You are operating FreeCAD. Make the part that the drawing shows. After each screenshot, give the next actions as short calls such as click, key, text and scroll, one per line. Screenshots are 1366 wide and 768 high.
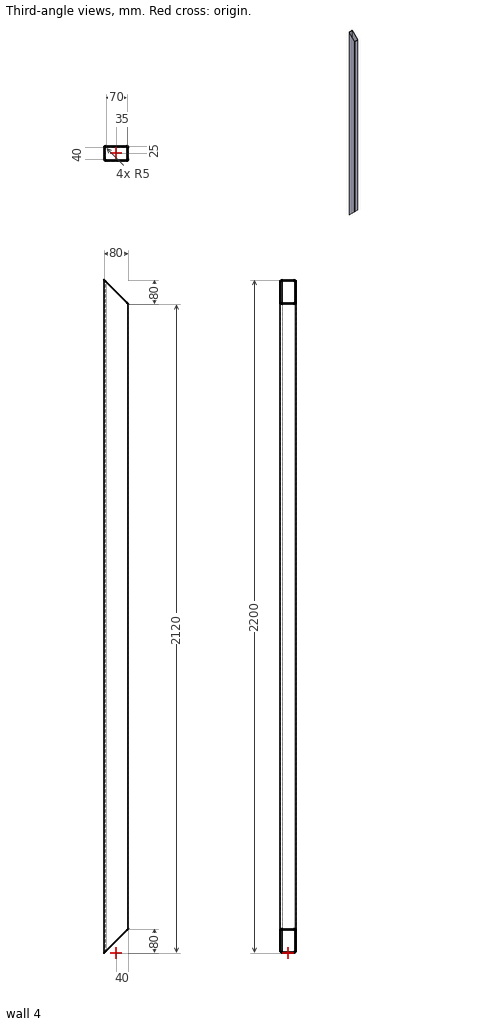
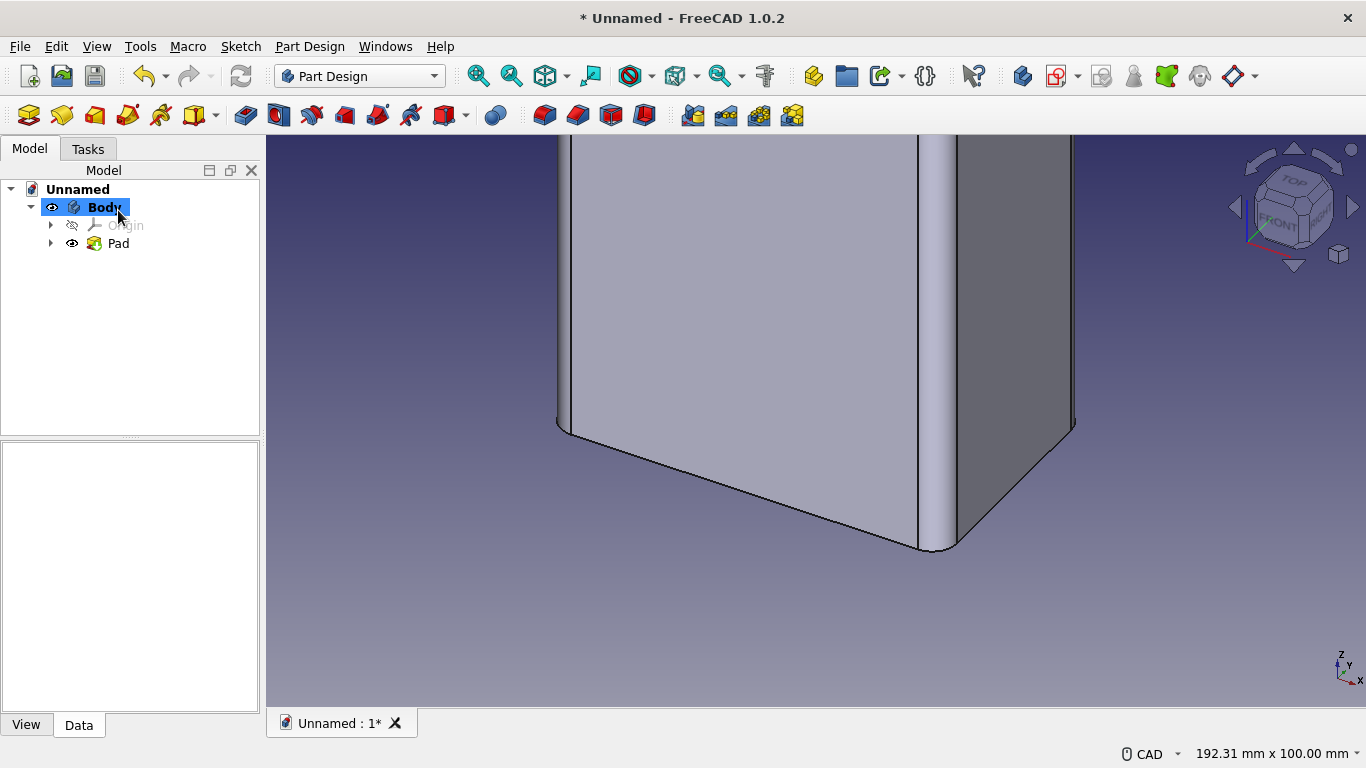
click(479, 76)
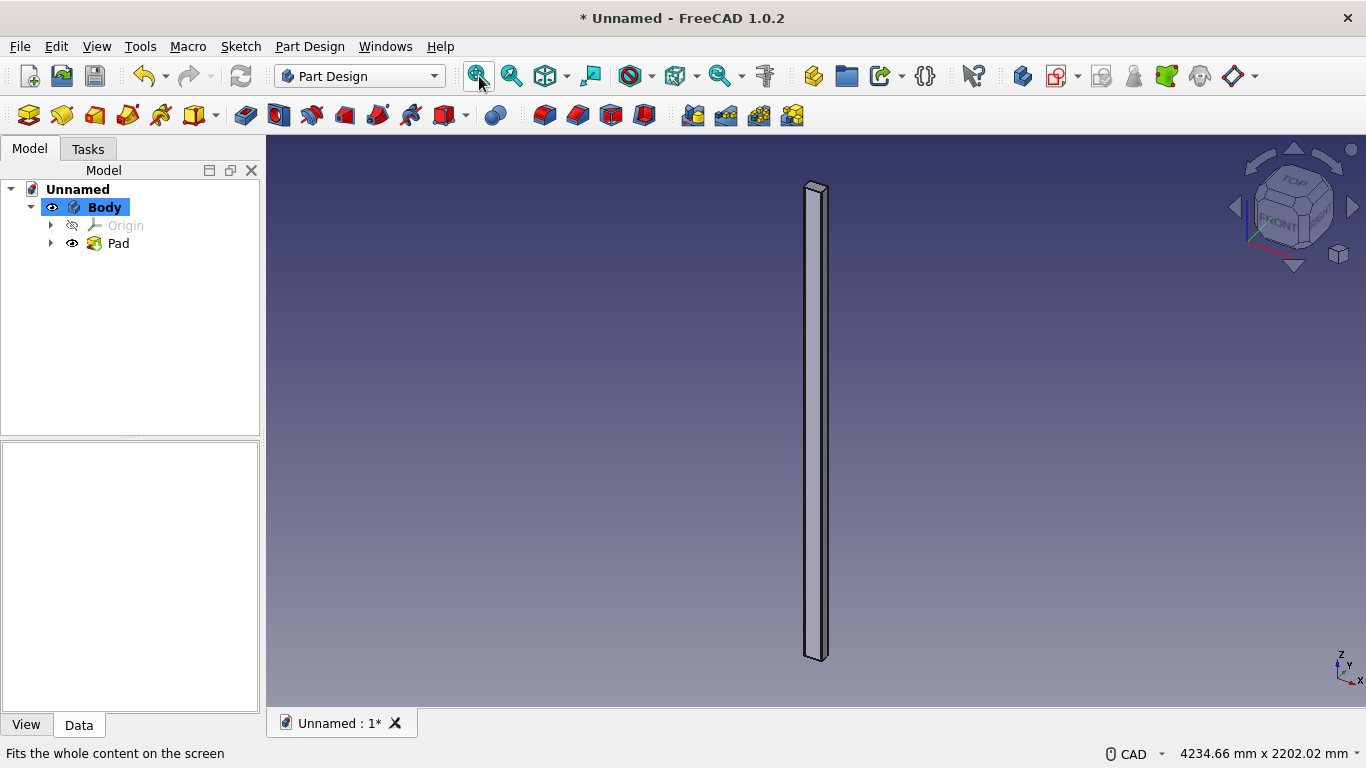
scroll(819, 187, up, 4)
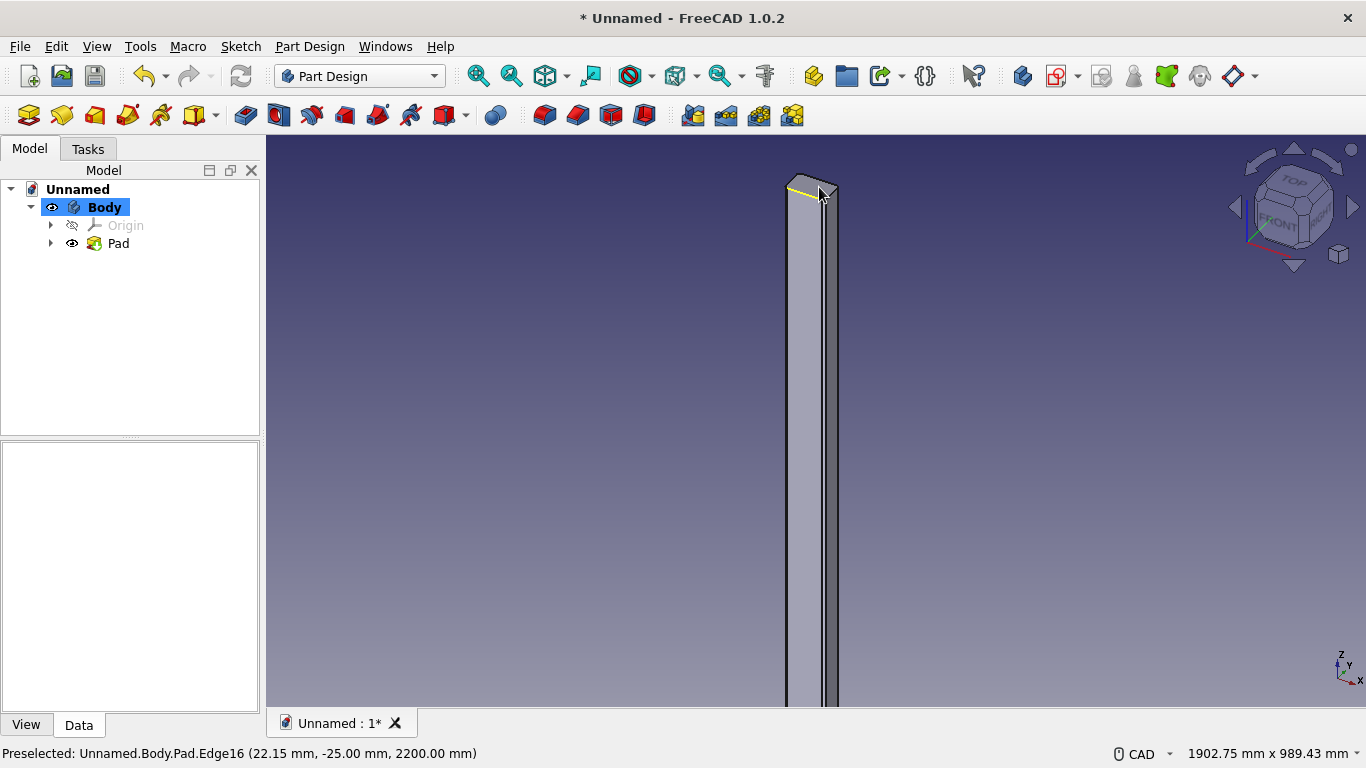
click(812, 186)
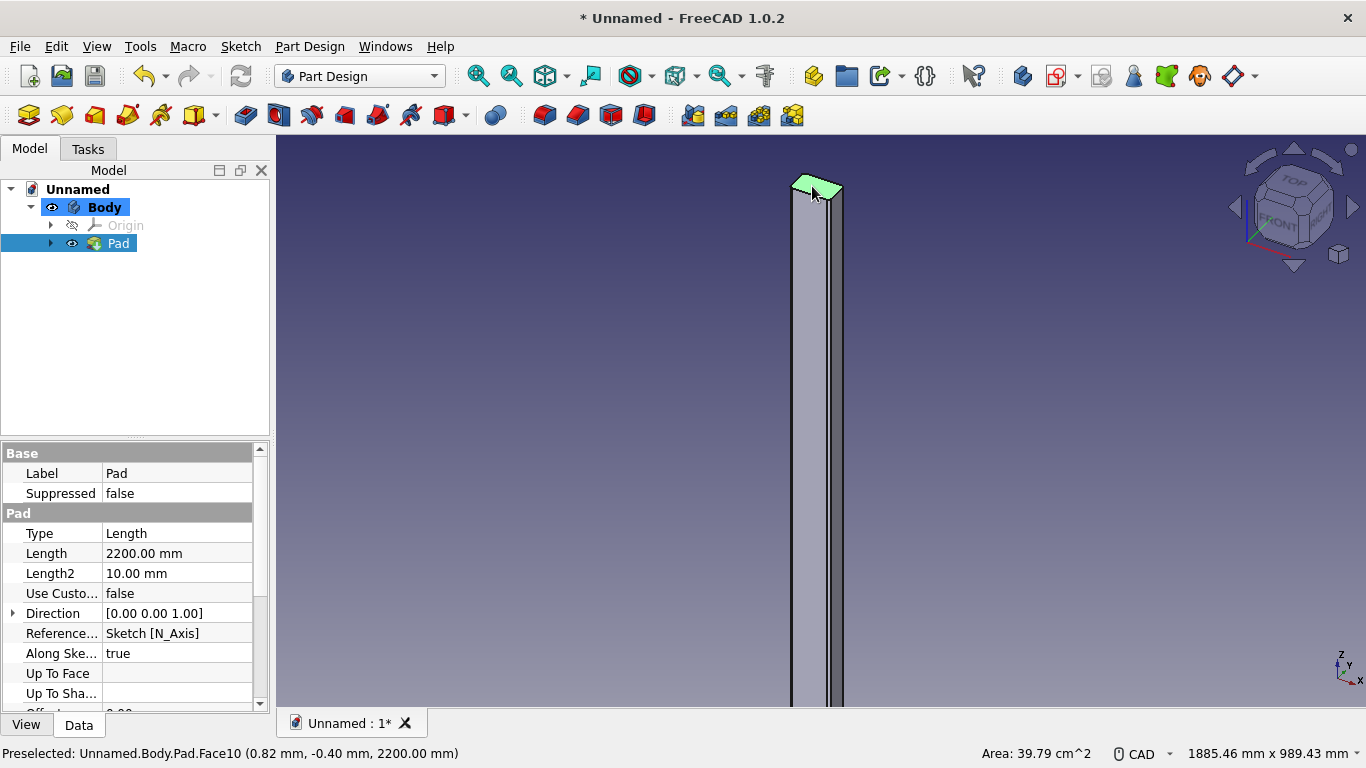
click(479, 76)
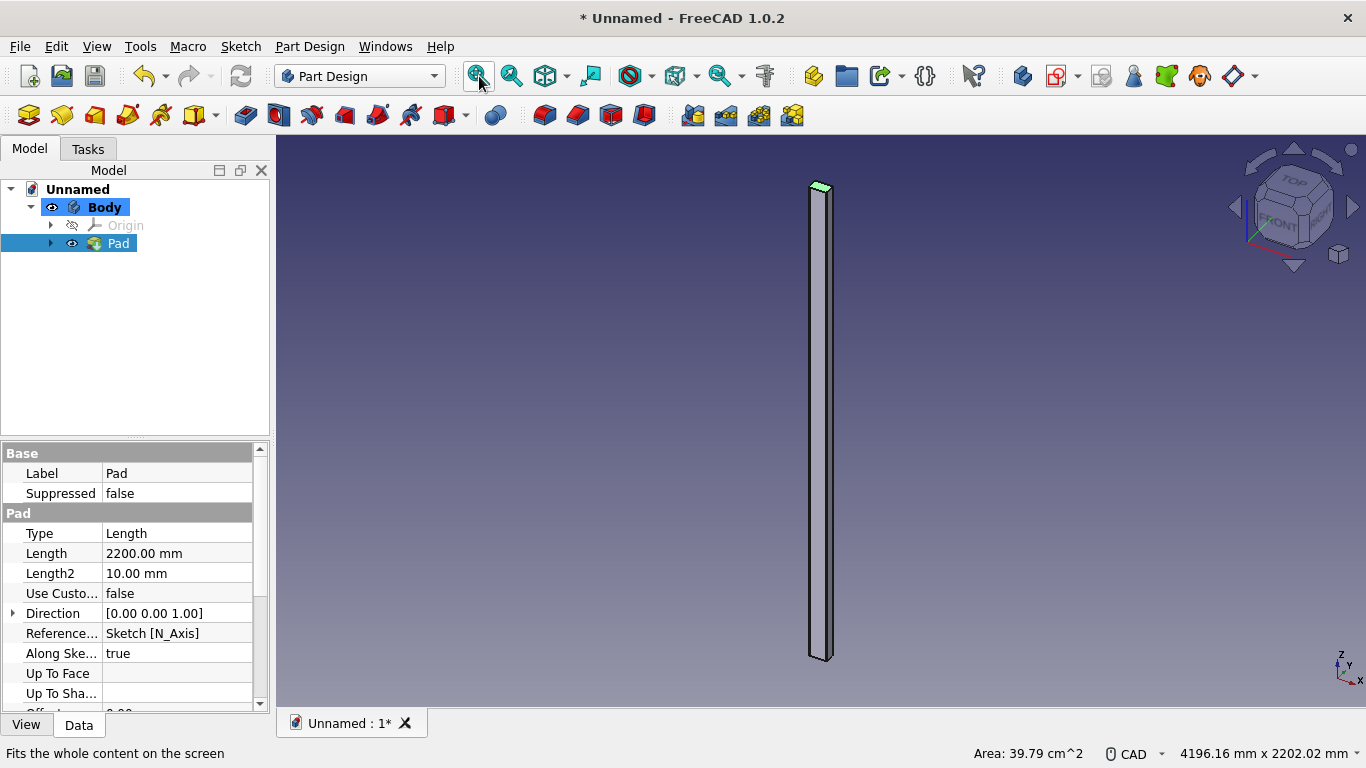
key(0)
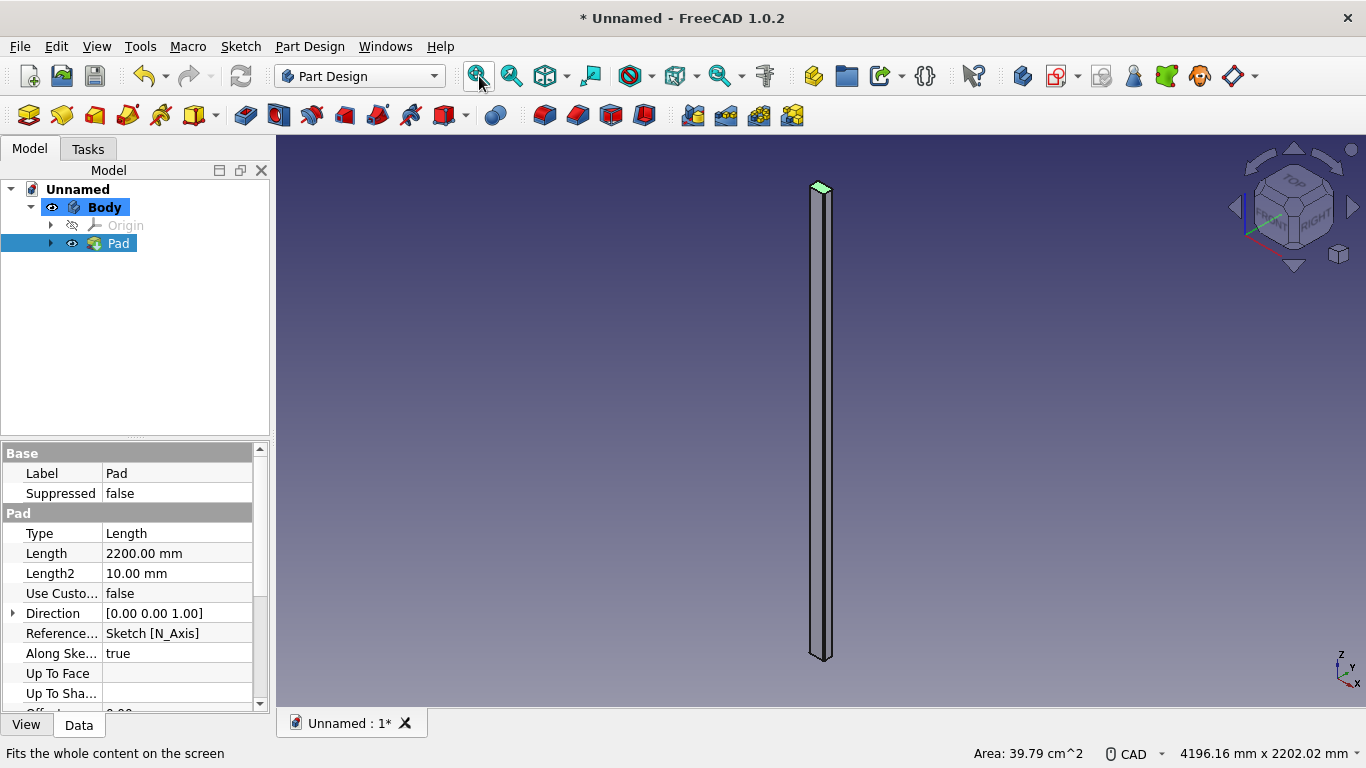
scroll(823, 655, up, 4)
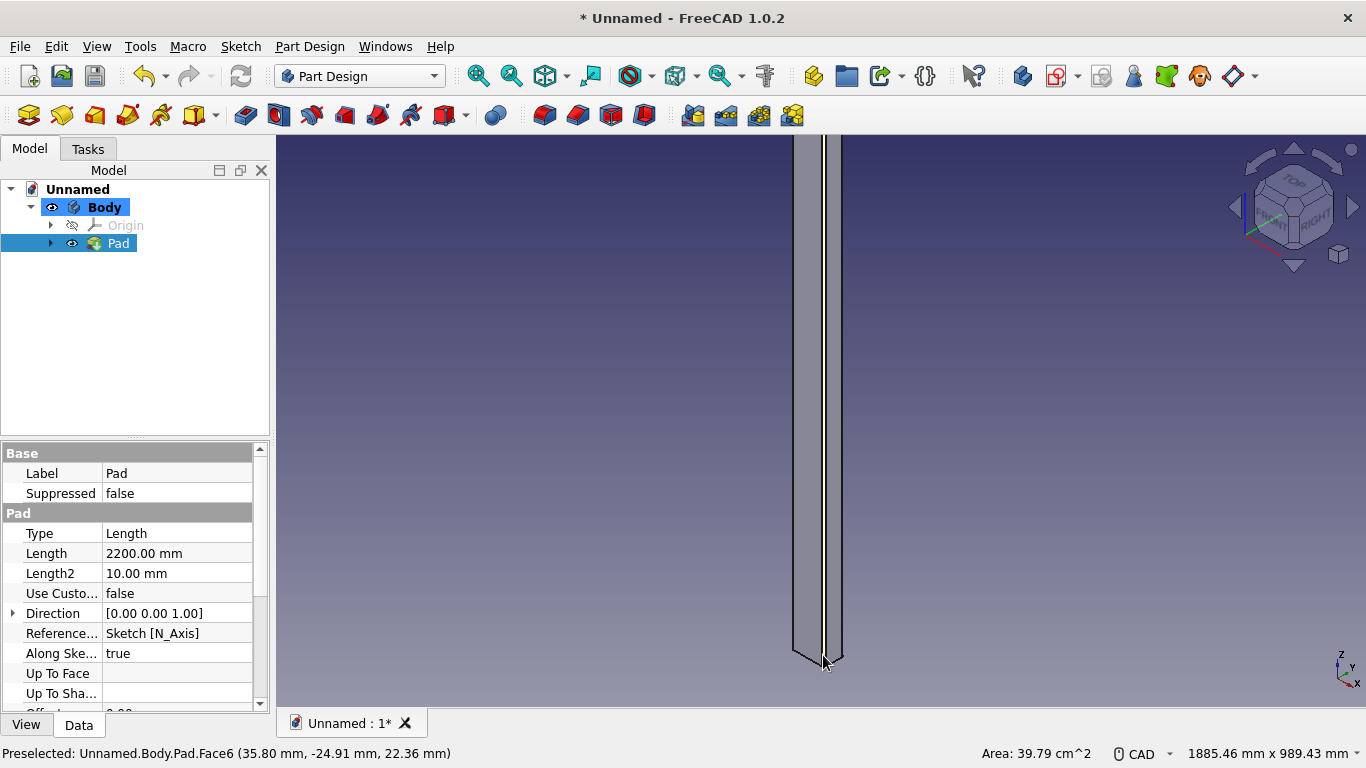
click(479, 76)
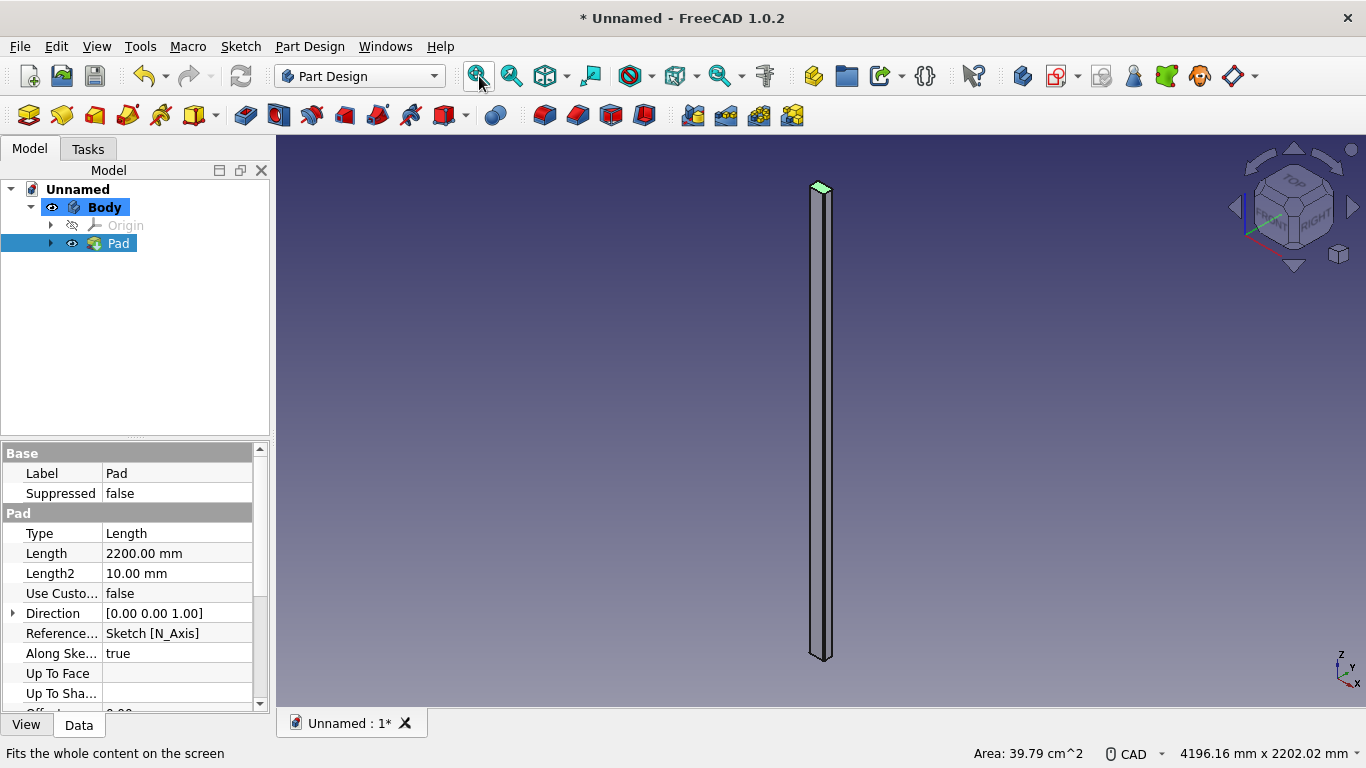
key(2)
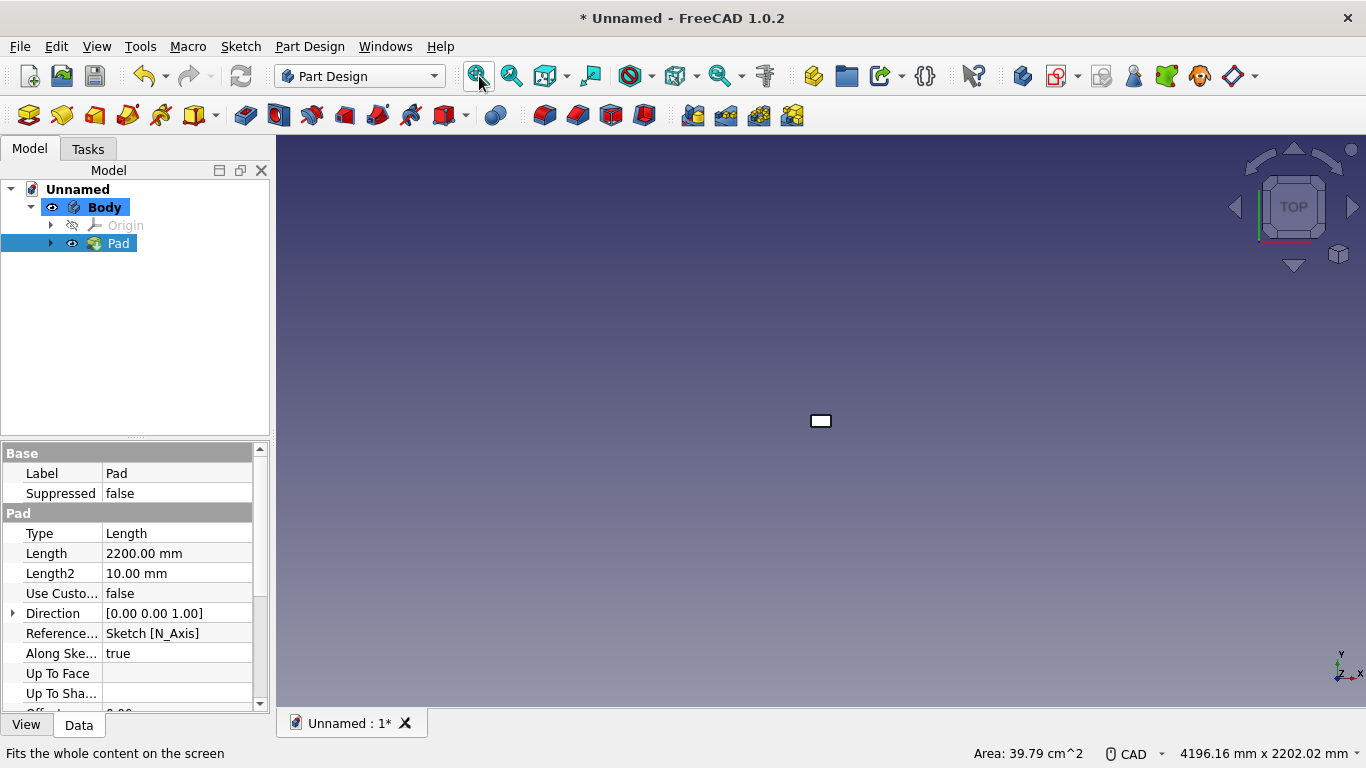
click(479, 76)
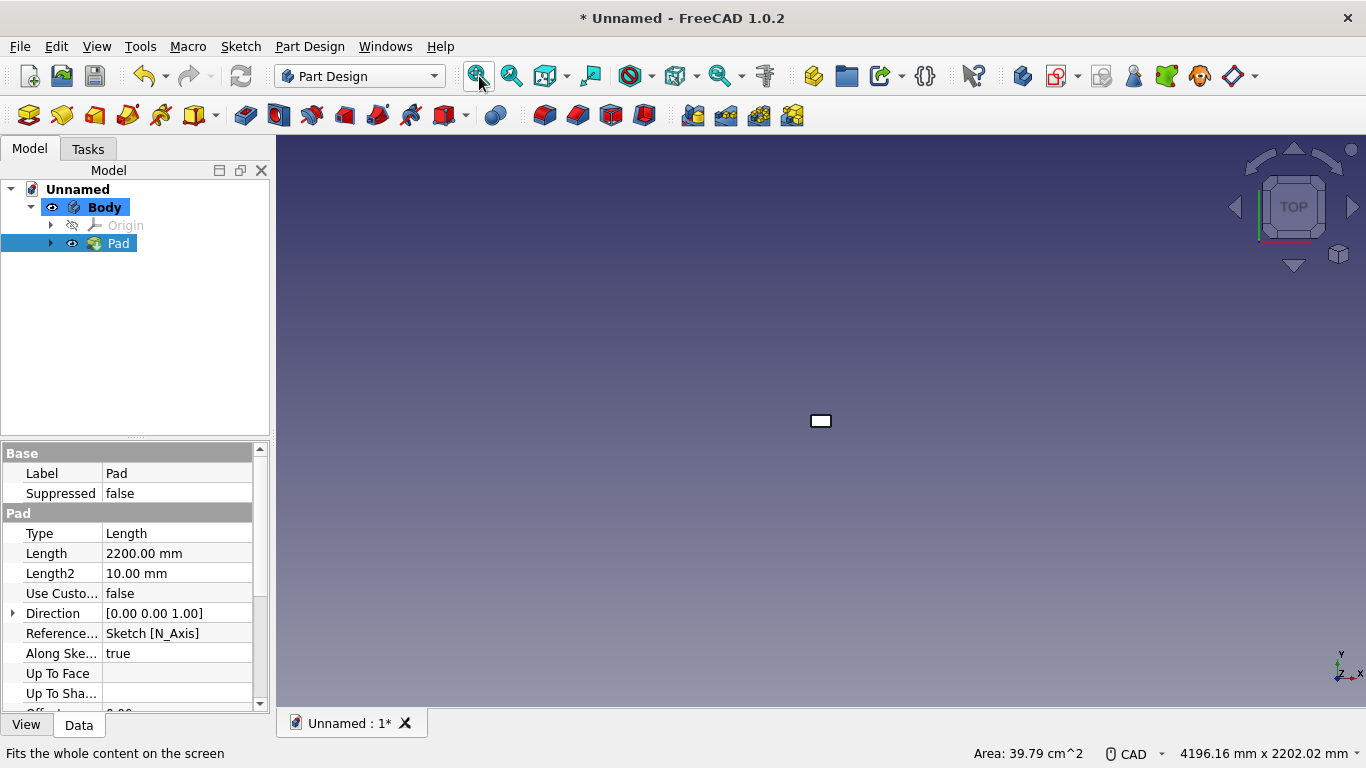
scroll(824, 420, up, 4)